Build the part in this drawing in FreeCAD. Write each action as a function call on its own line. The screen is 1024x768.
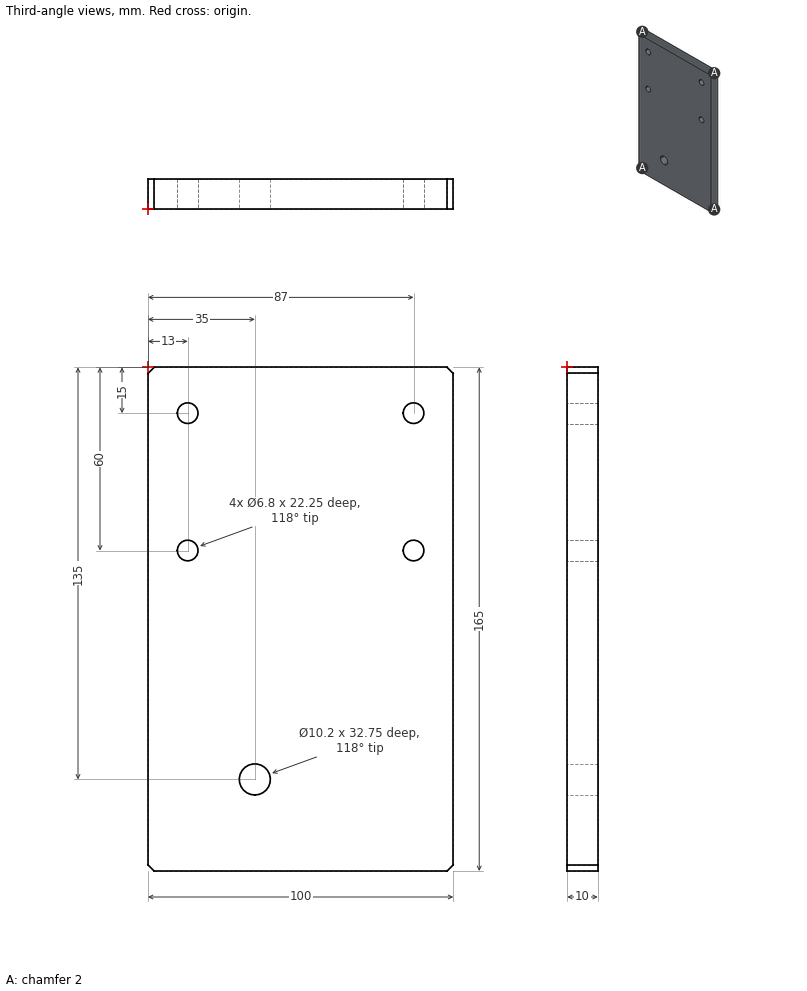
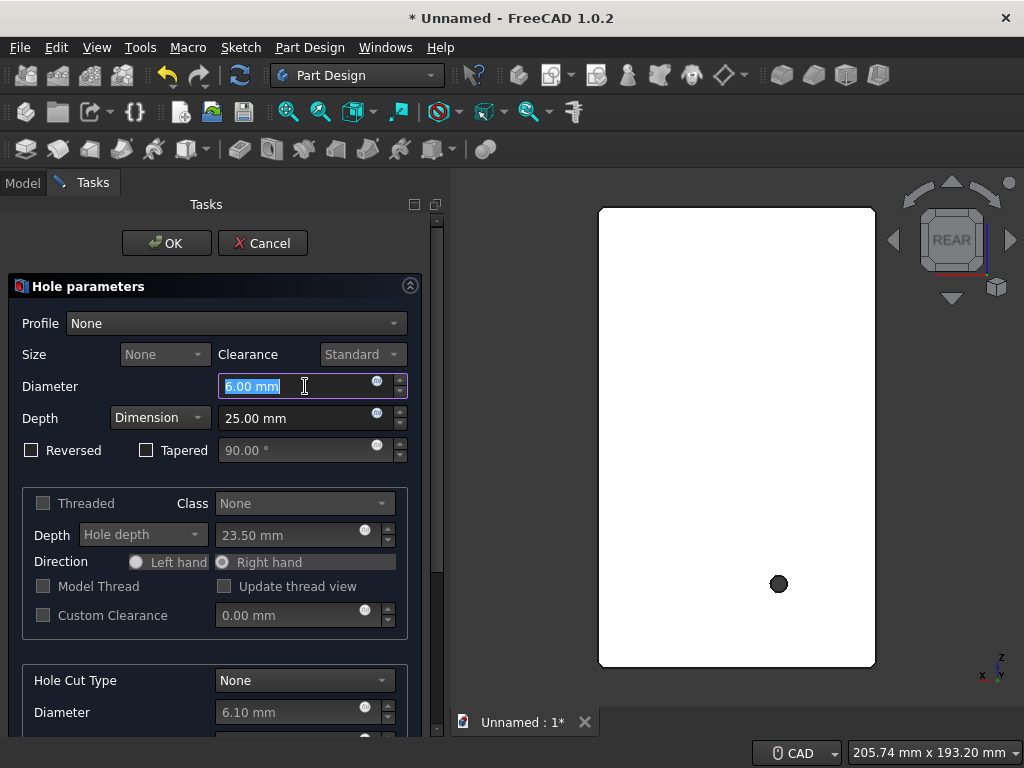
text(10.2)
key(Tab)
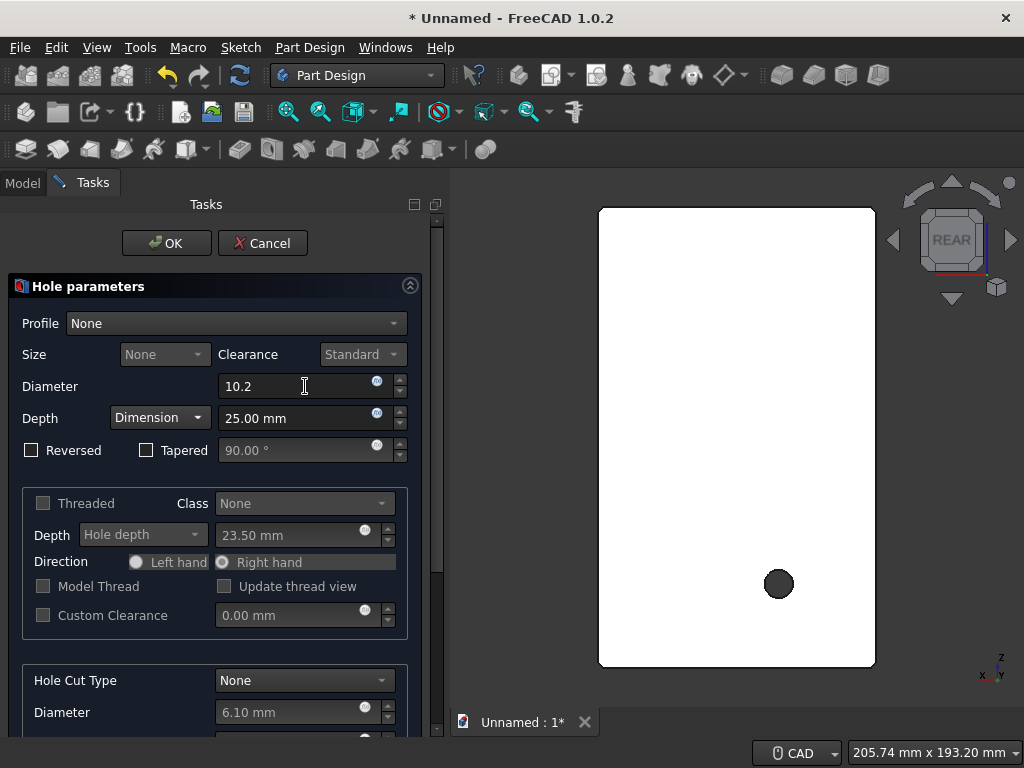
triple_click(305, 418)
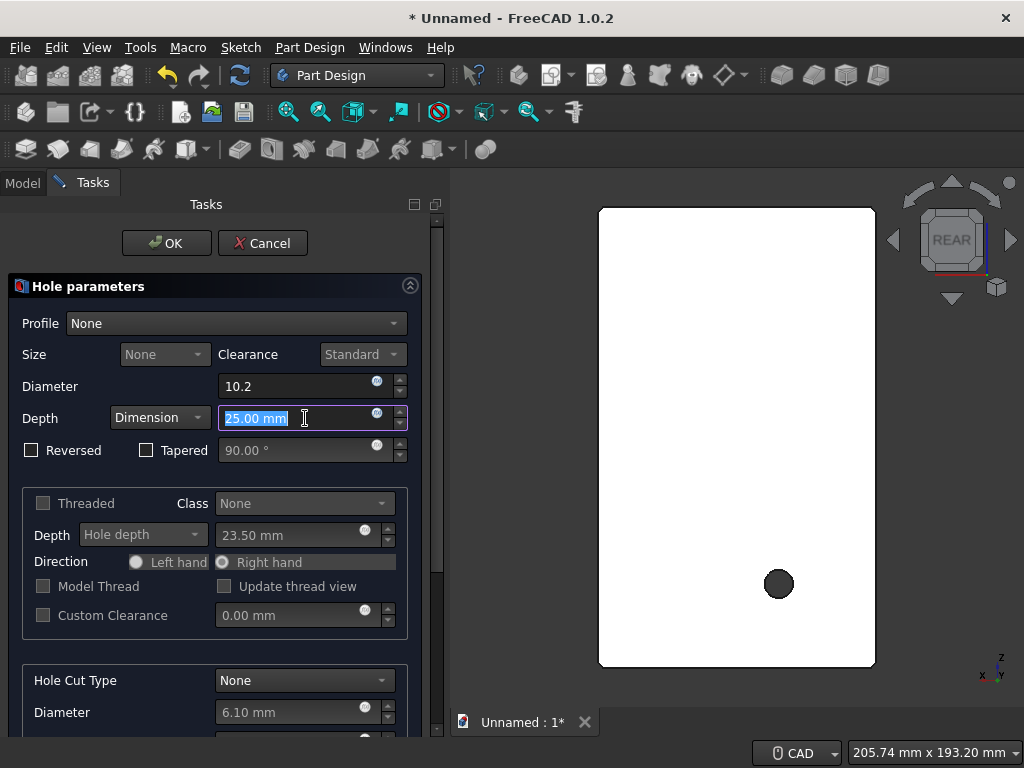
text(32.75)
key(Tab)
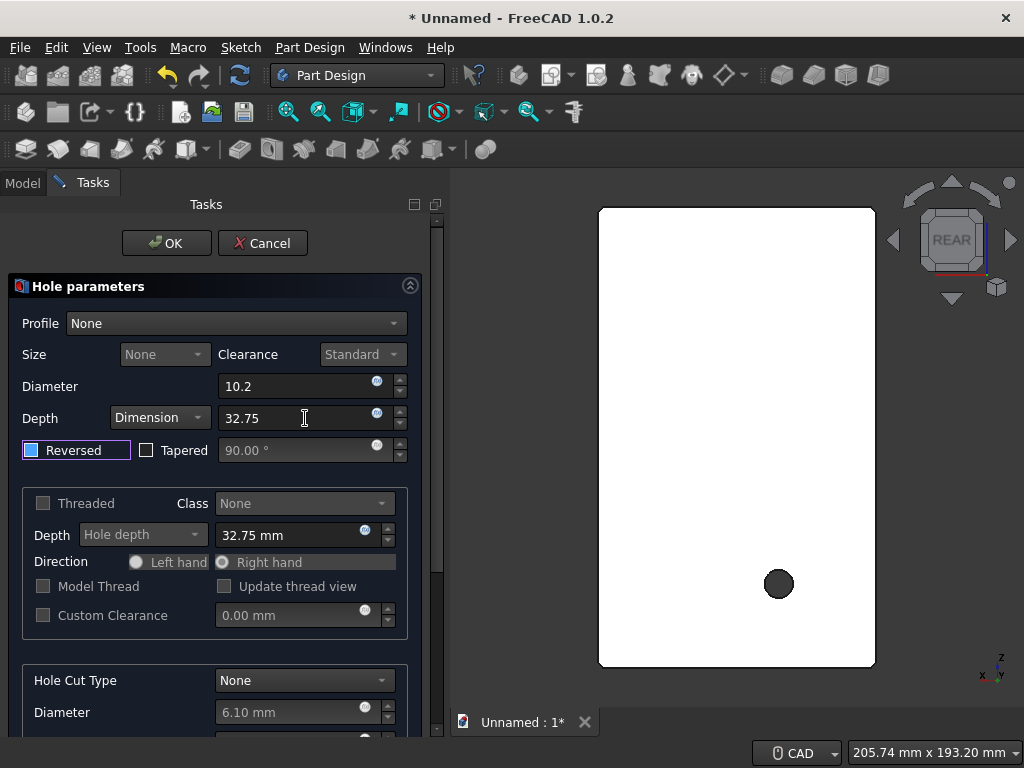
click(167, 243)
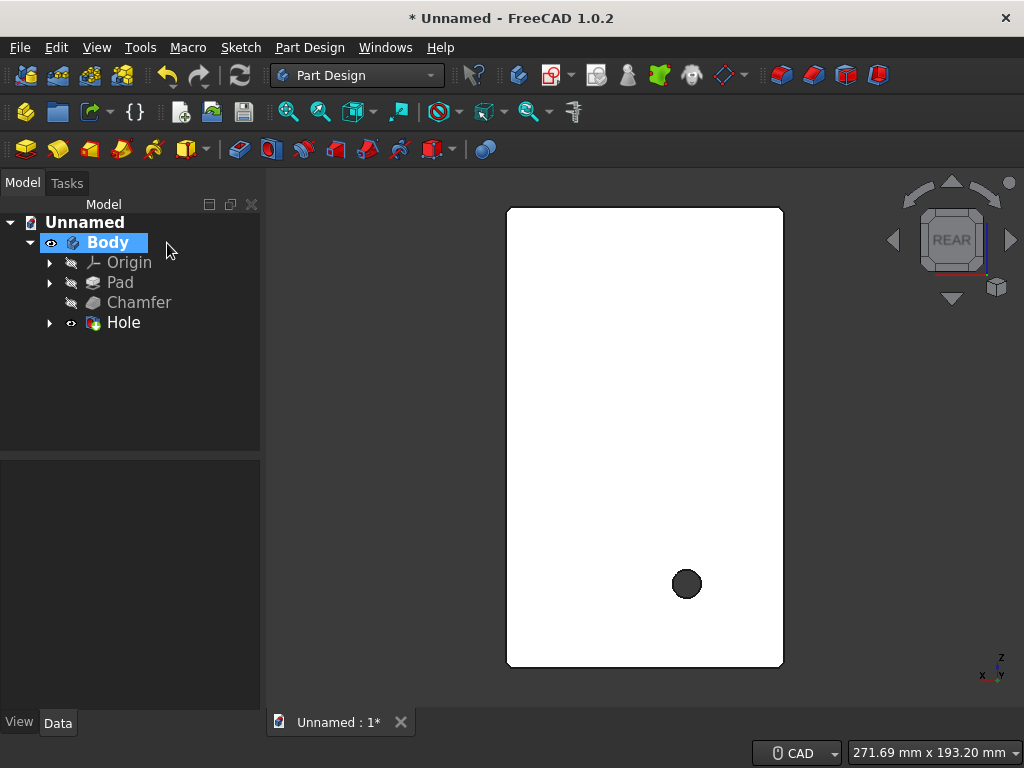
click(645, 371)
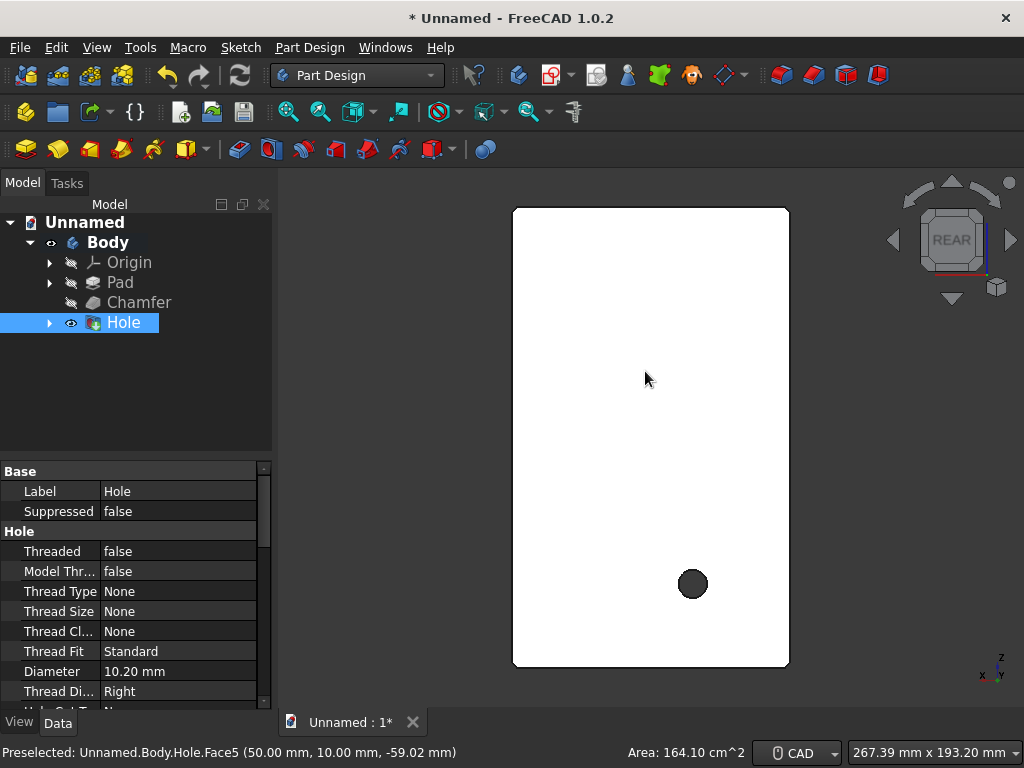
click(552, 76)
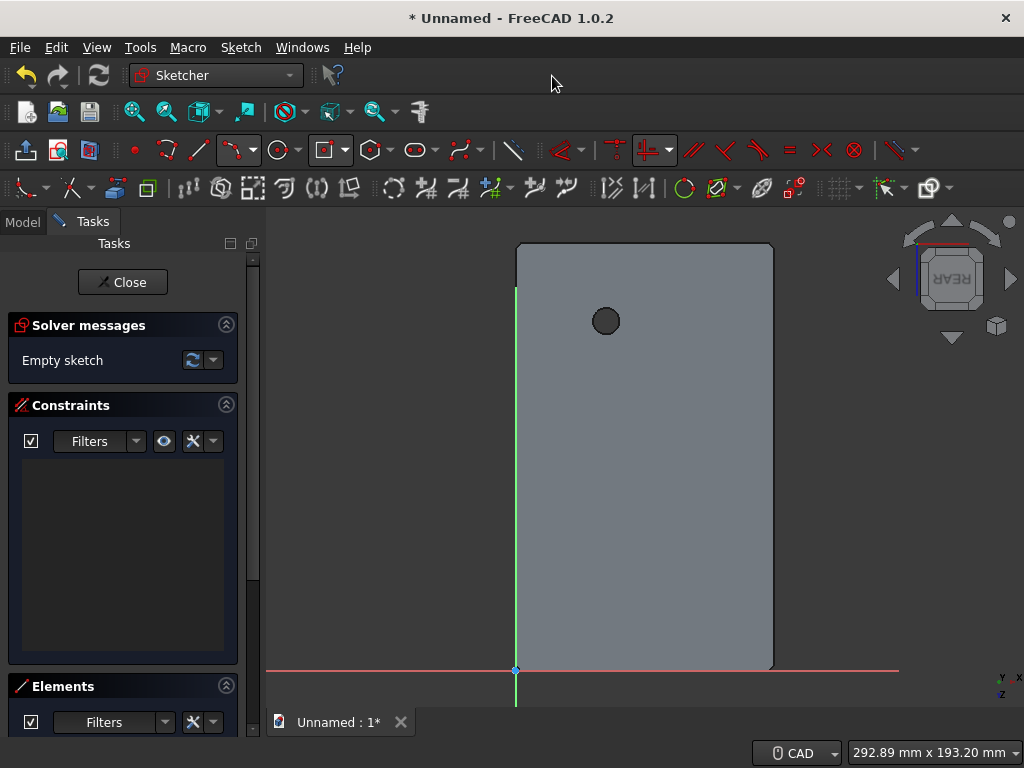
scroll(576, 457, down, 5)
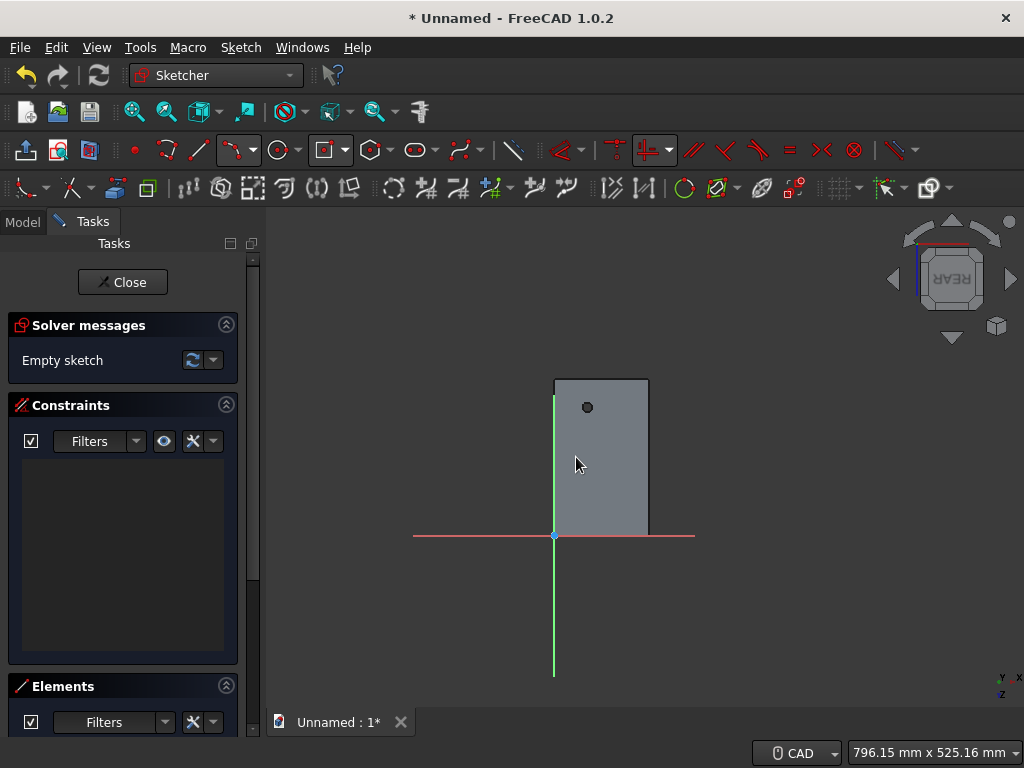
scroll(602, 518, up, 8)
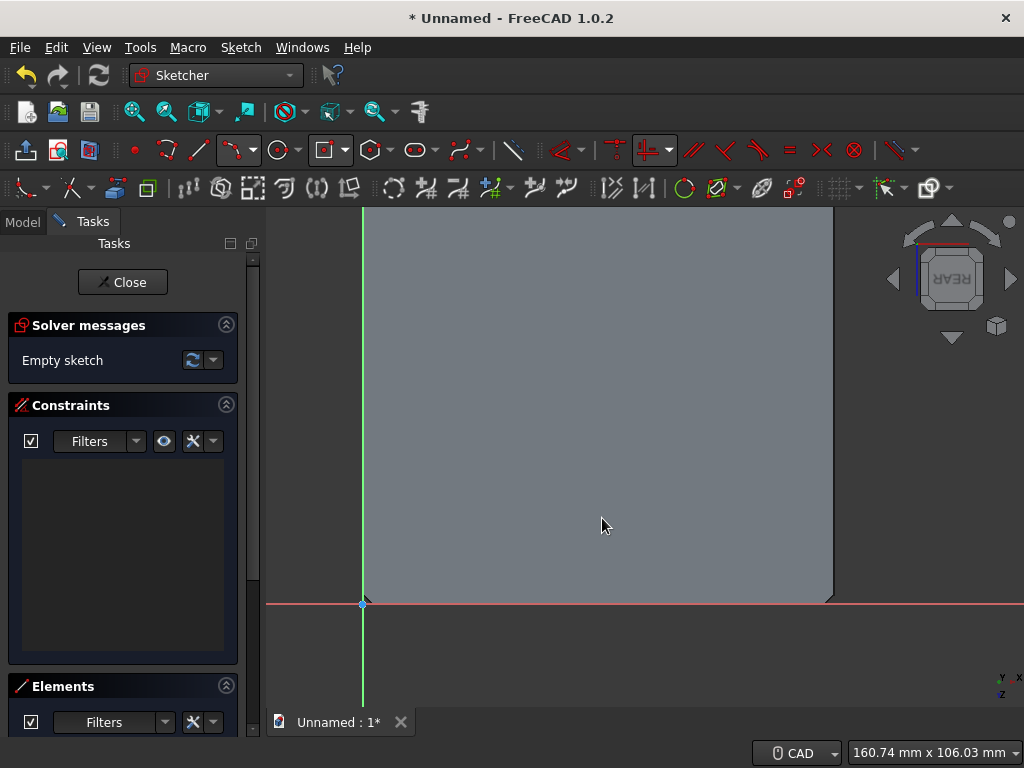
click(278, 150)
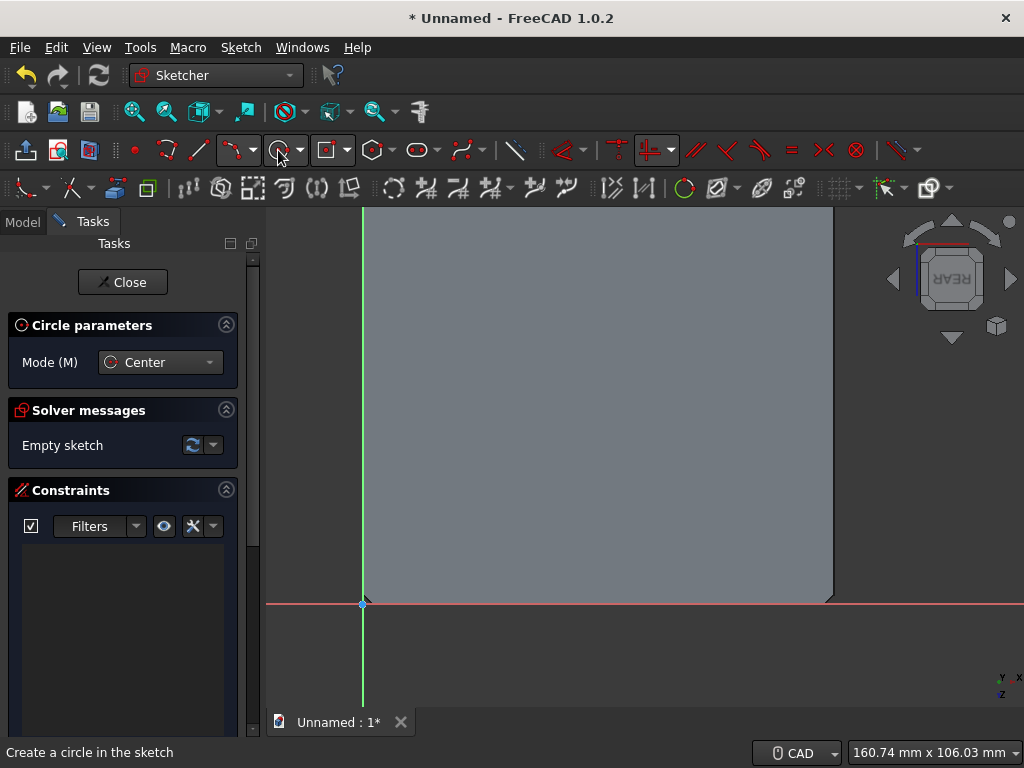
scroll(424, 321, up, 2)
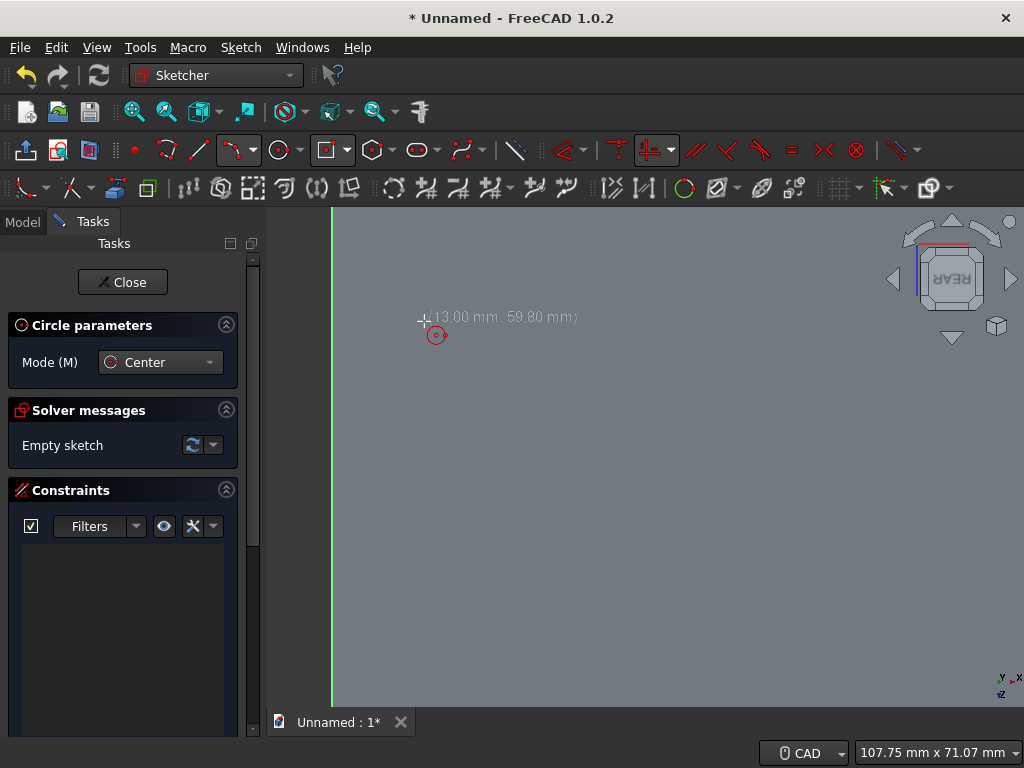
click(424, 321)
move(441, 304)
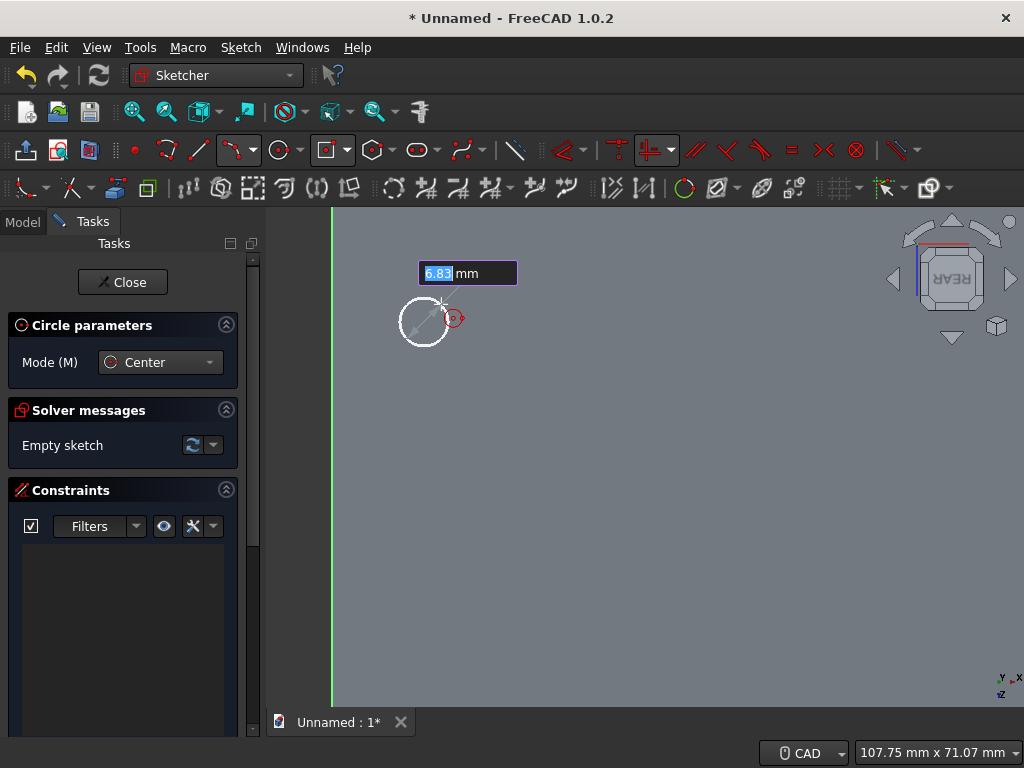
text(6.8)
key(Return)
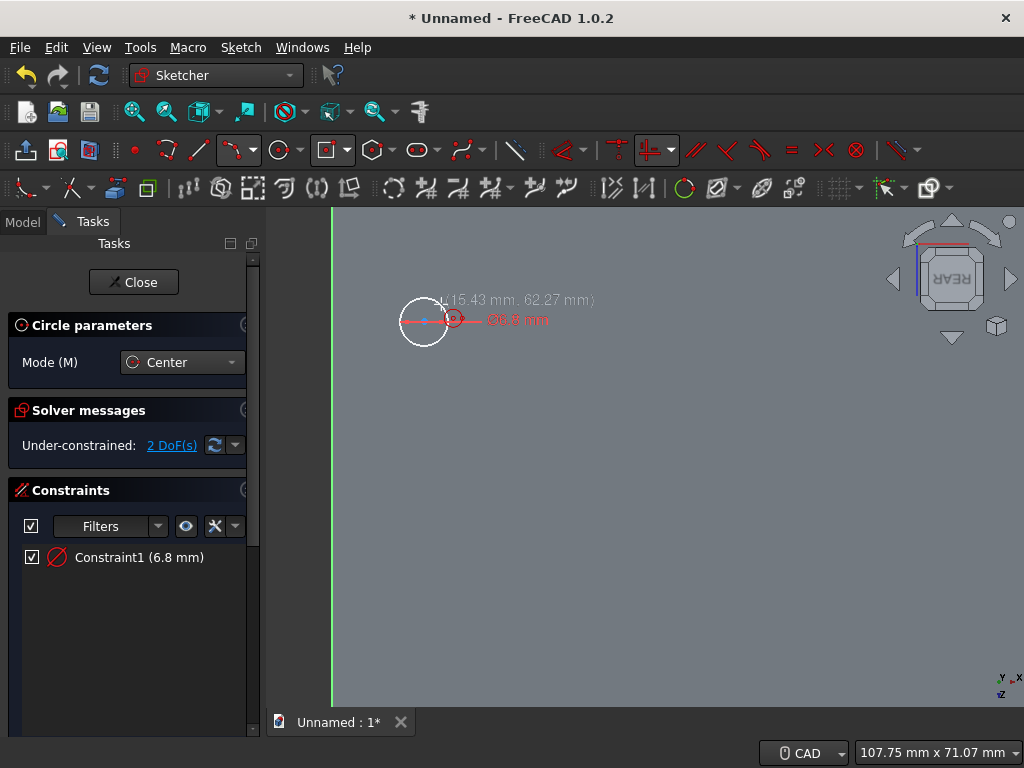
click(424, 638)
move(441, 621)